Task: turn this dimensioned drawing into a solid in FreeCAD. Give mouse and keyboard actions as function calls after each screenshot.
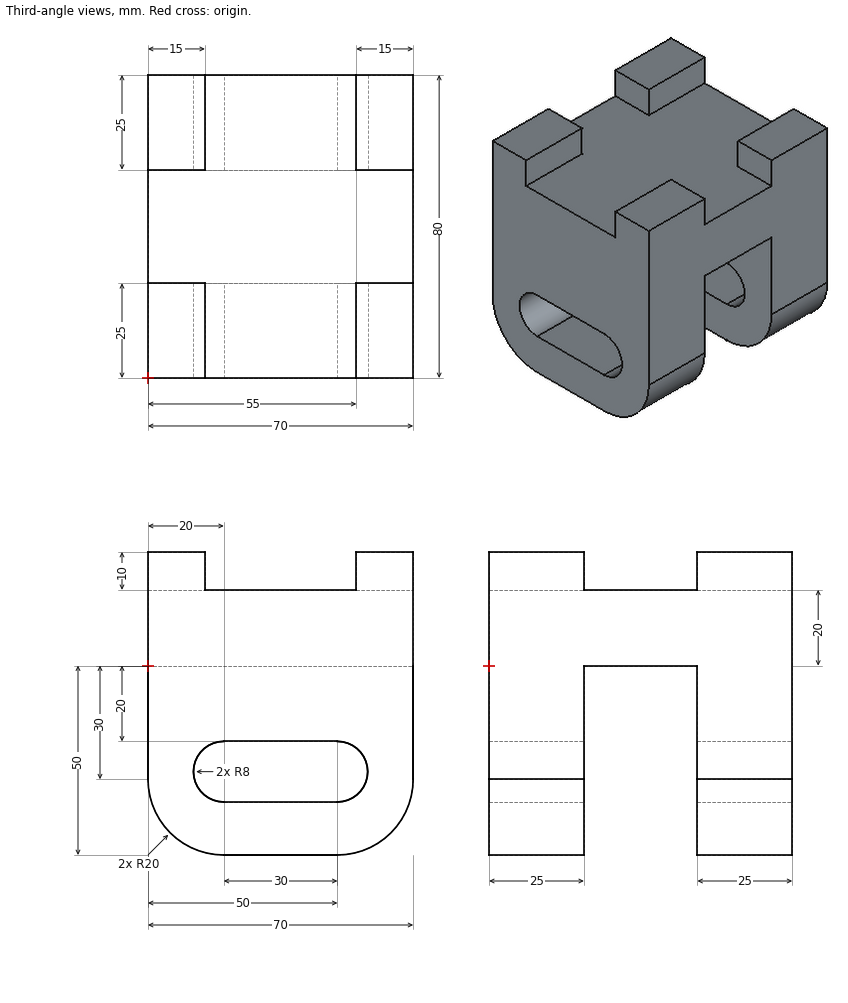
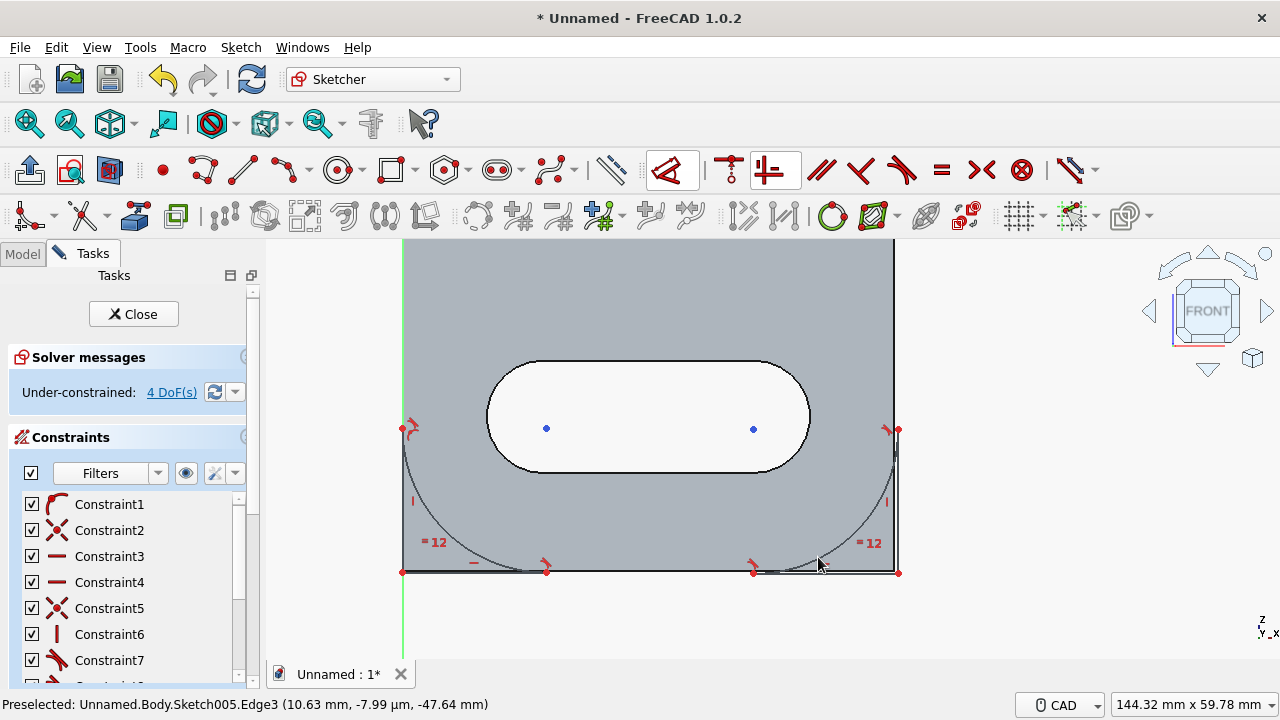
click(481, 557)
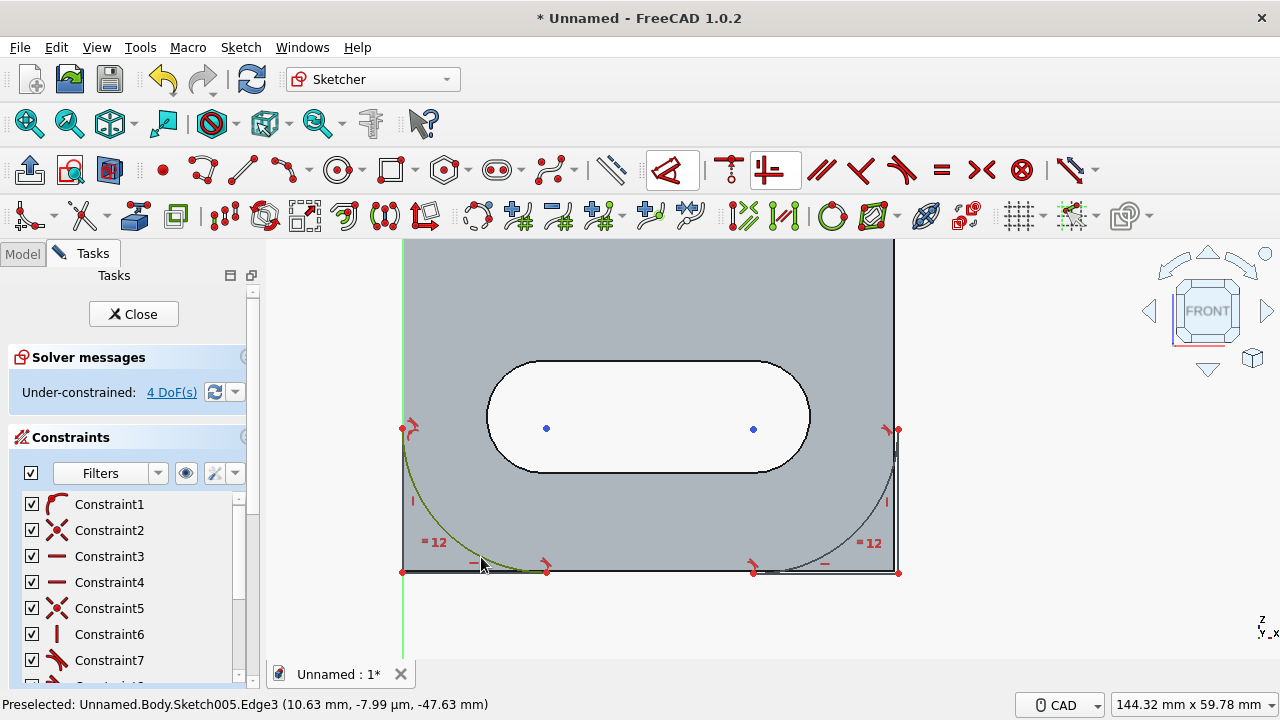
key(k)
key(r)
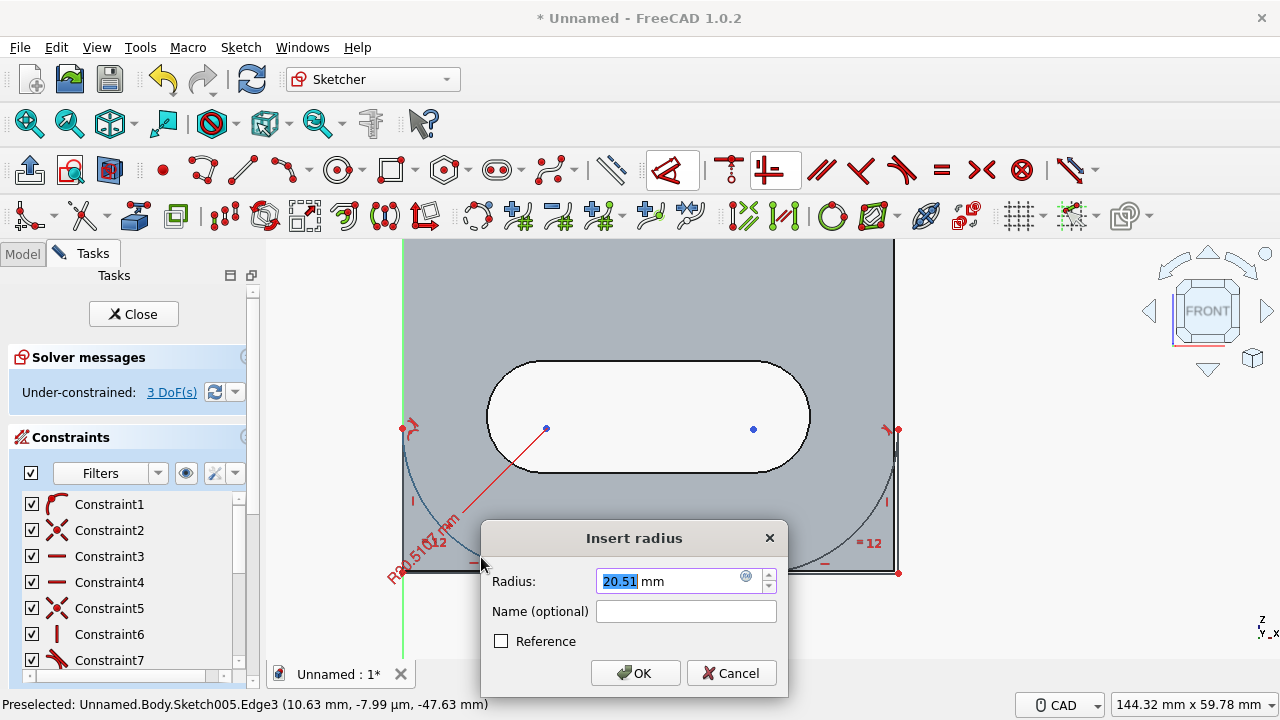
text(20)
key(Return)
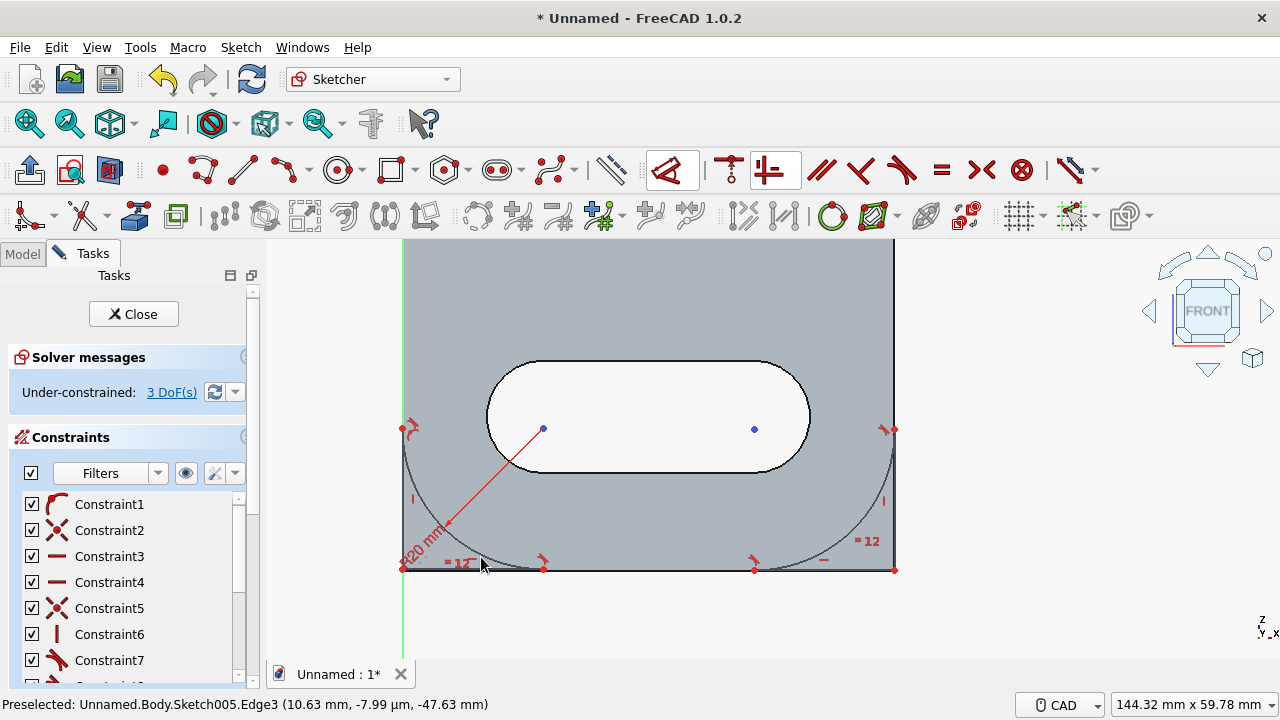
click(403, 429)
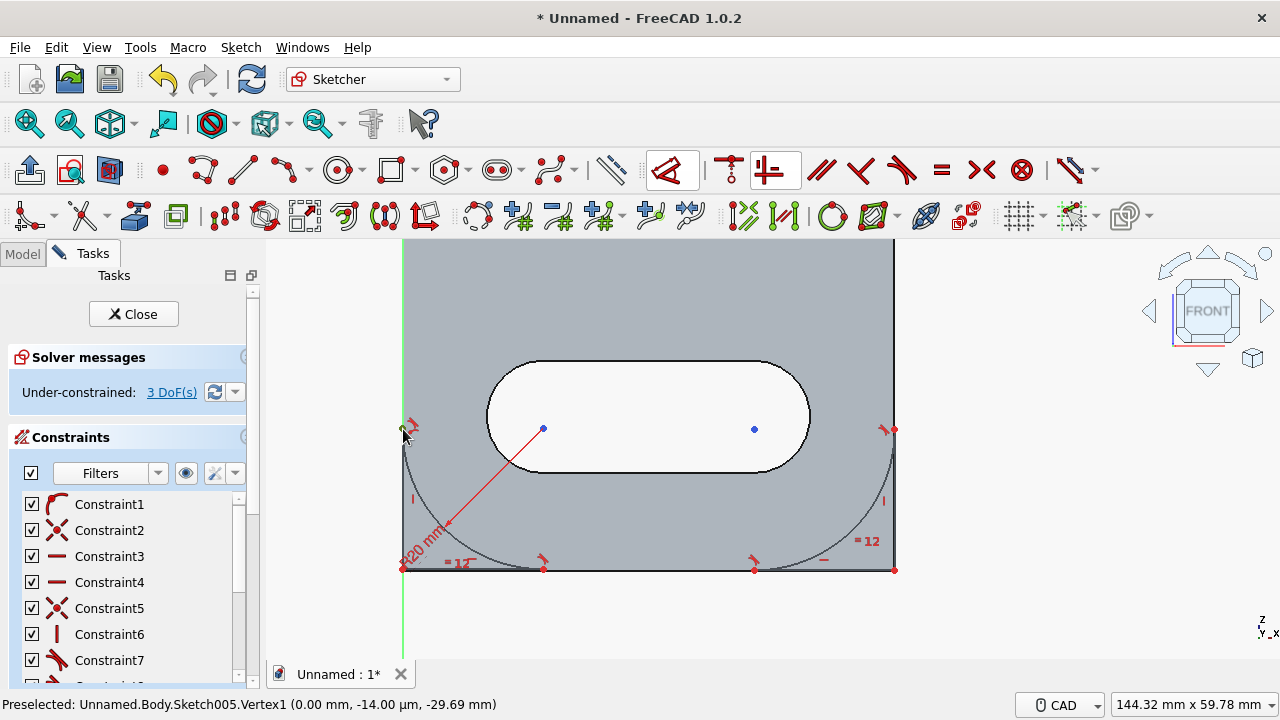
key(i)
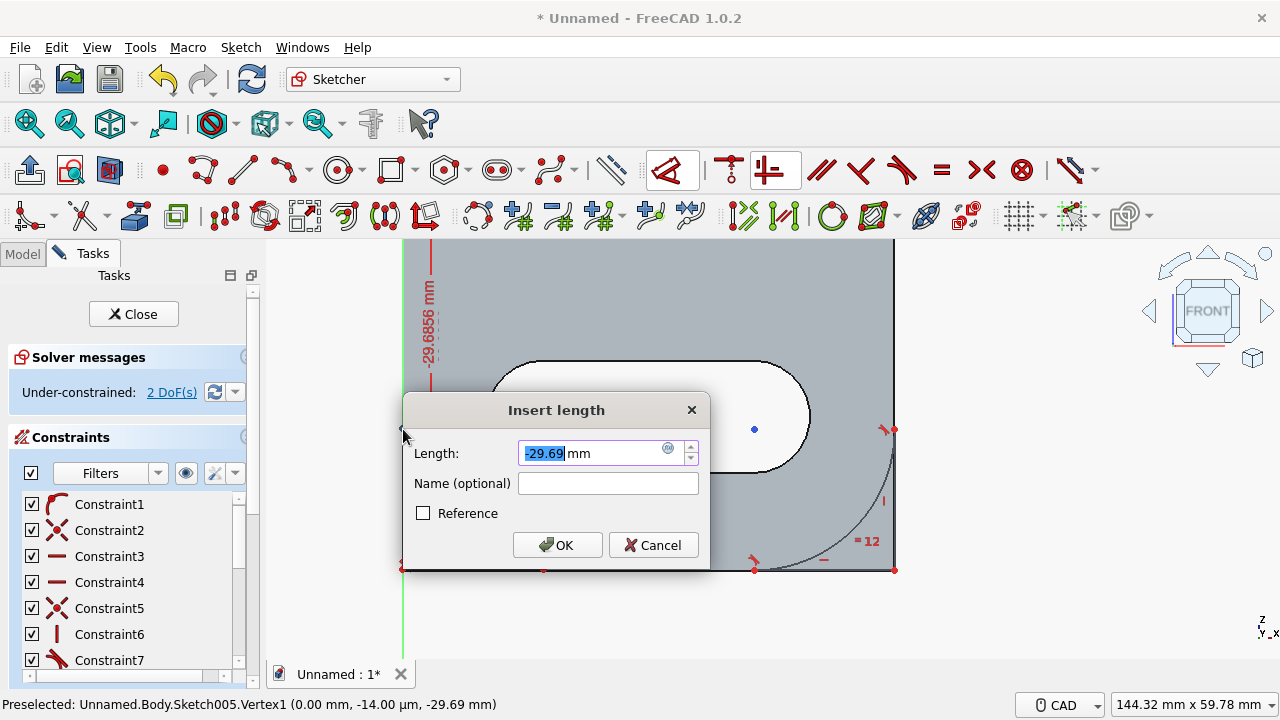
text(-30)
key(Return)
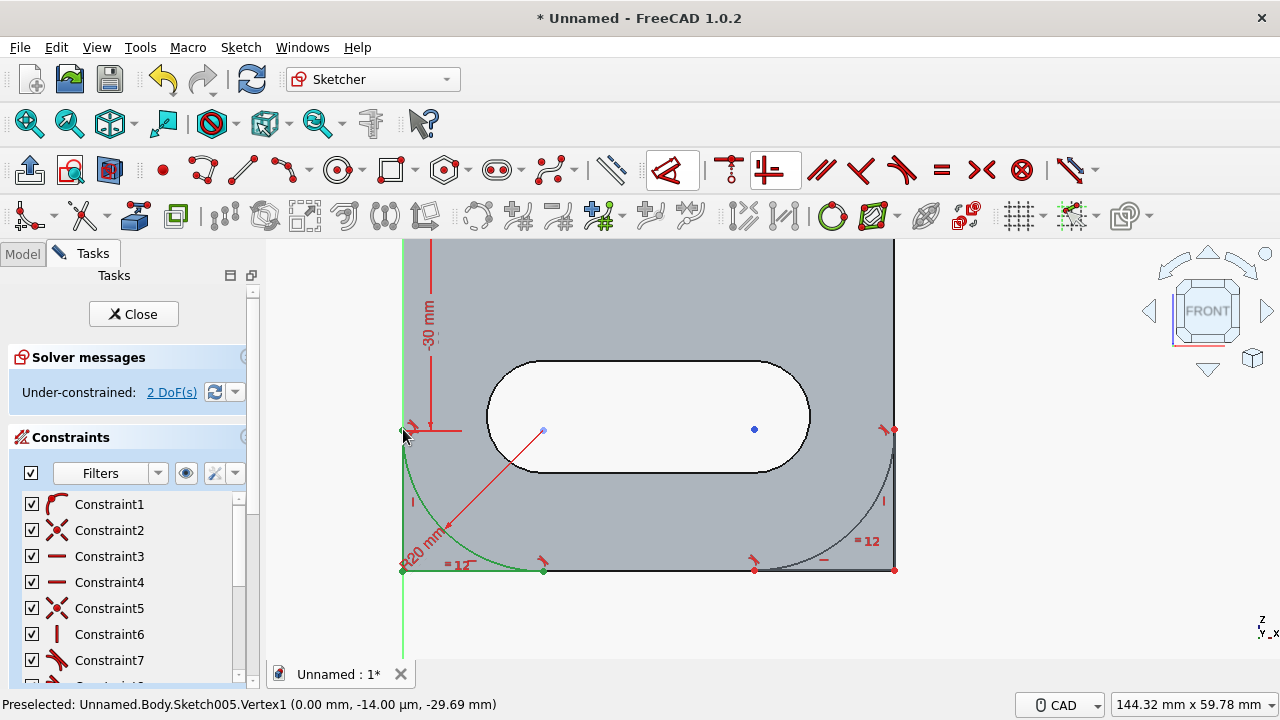
click(754, 570)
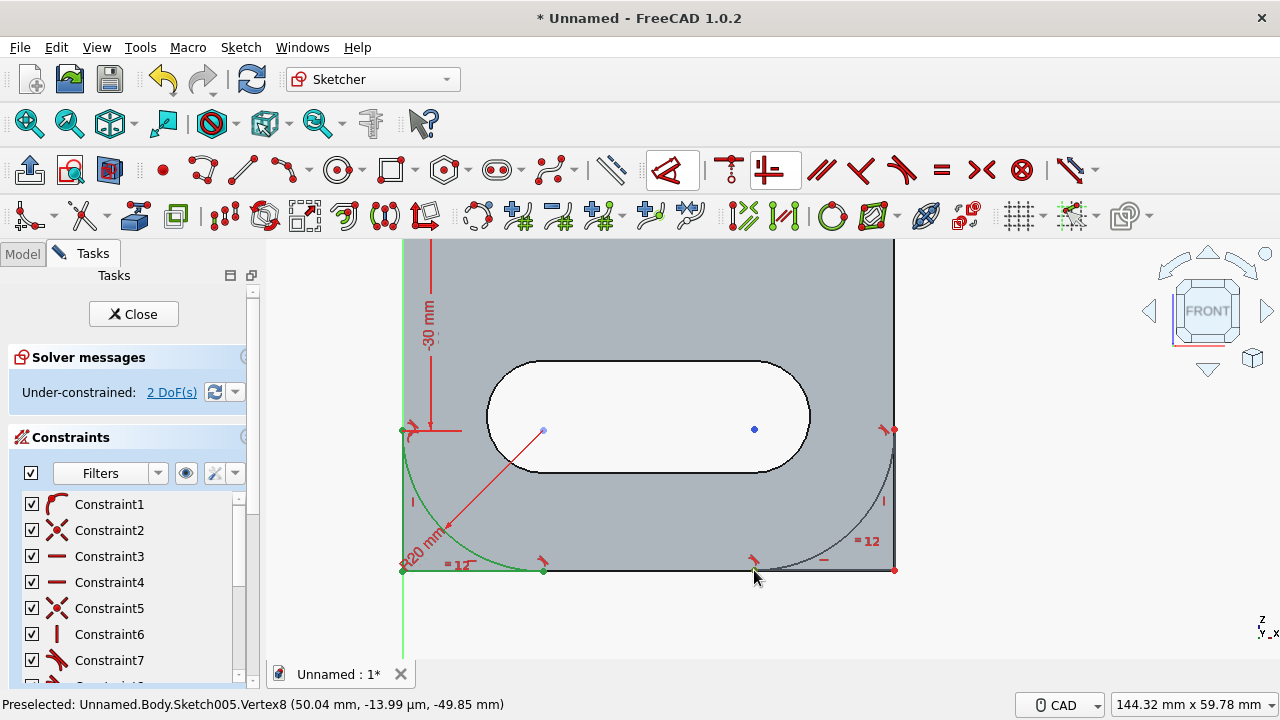
key(l)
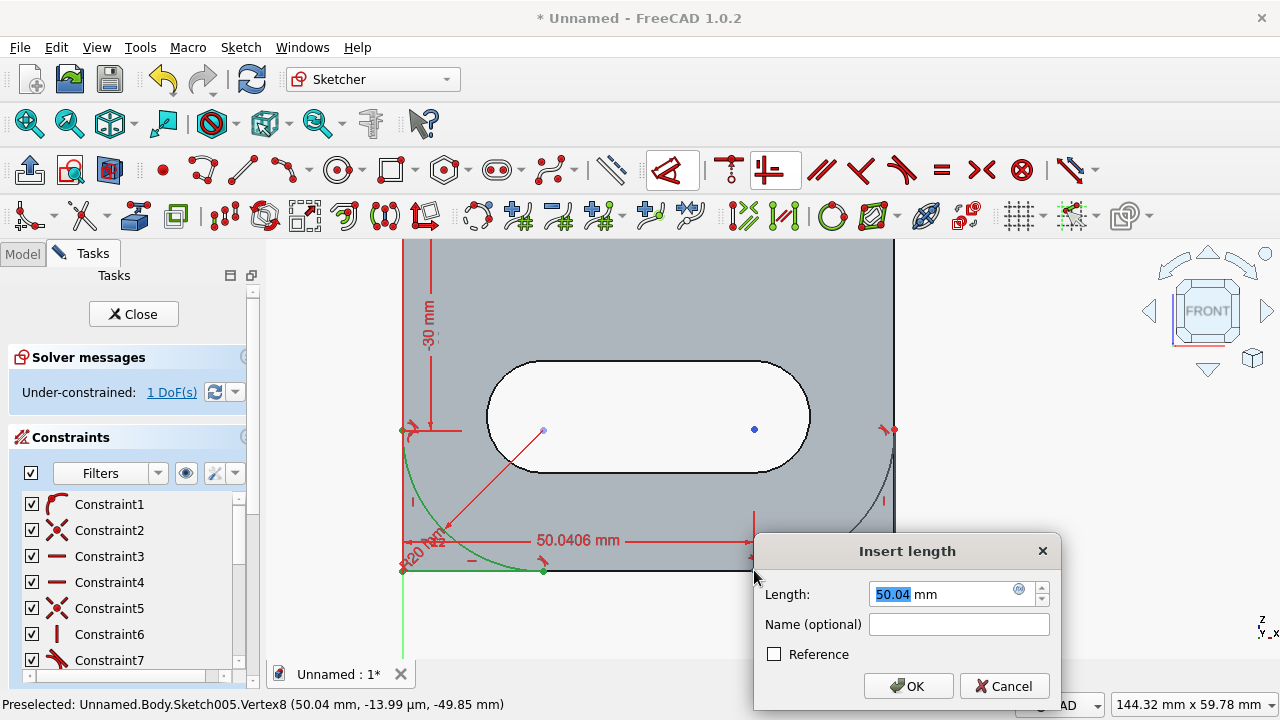
text(50)
key(Return)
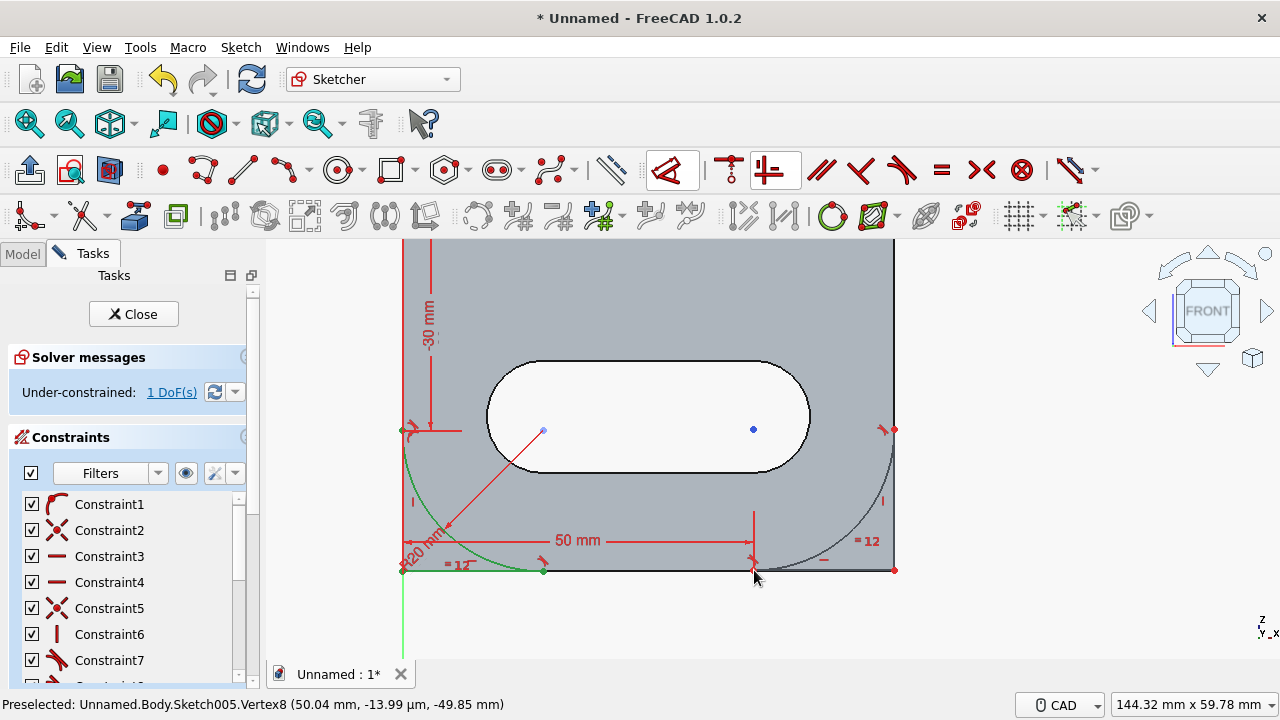
click(754, 570)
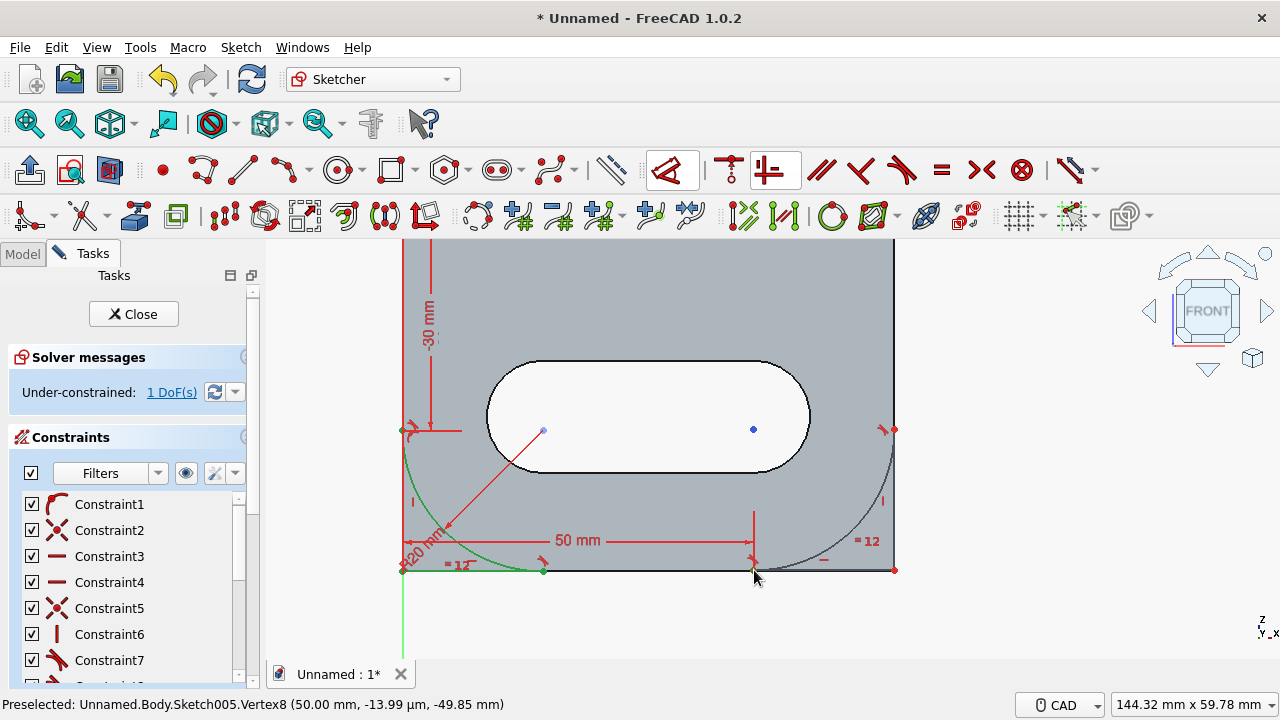
key(i)